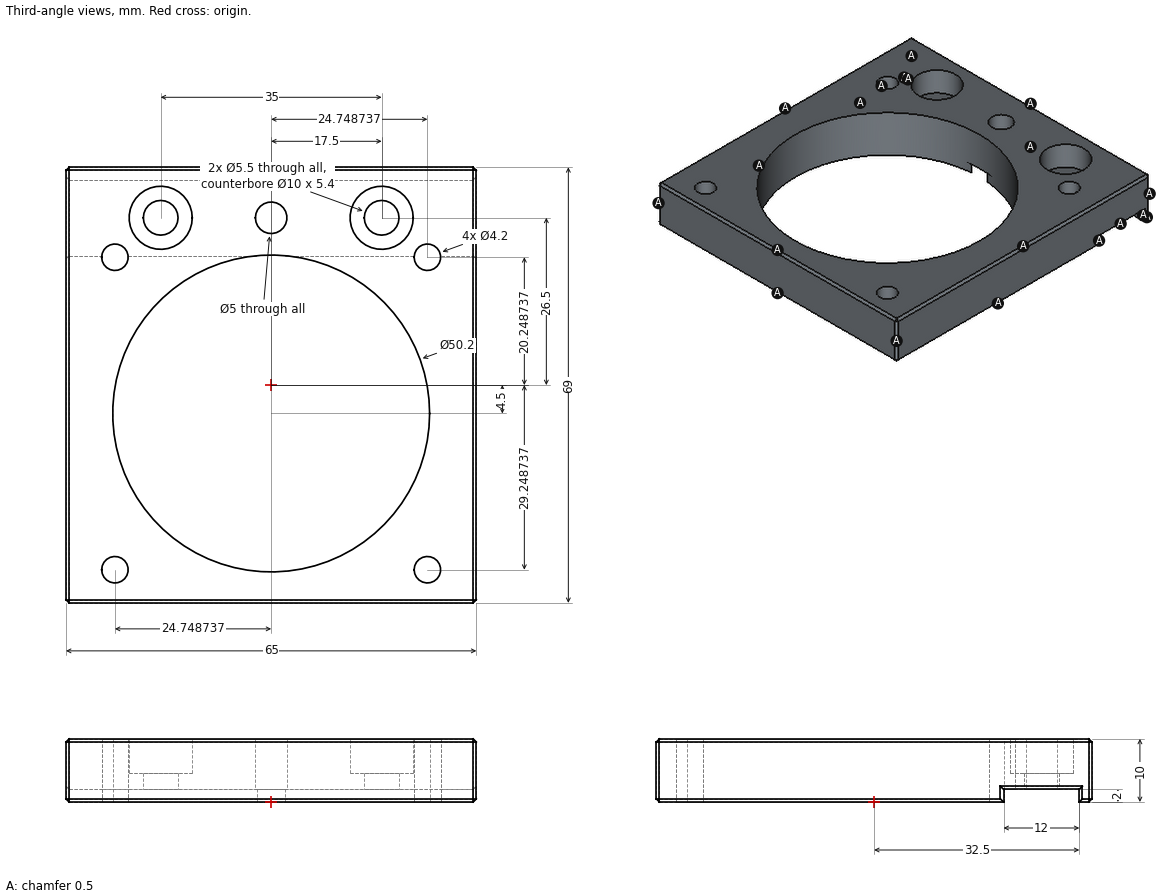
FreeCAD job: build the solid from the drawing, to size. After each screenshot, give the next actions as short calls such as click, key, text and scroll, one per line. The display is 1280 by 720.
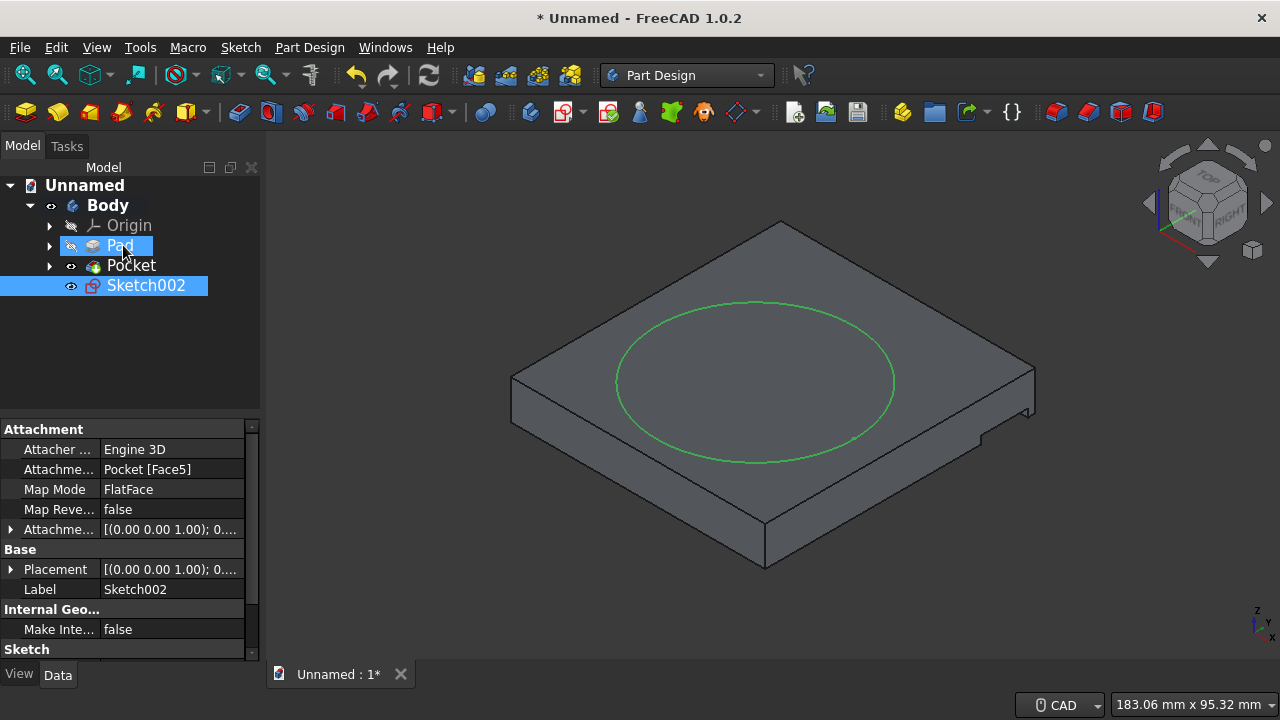
click(240, 112)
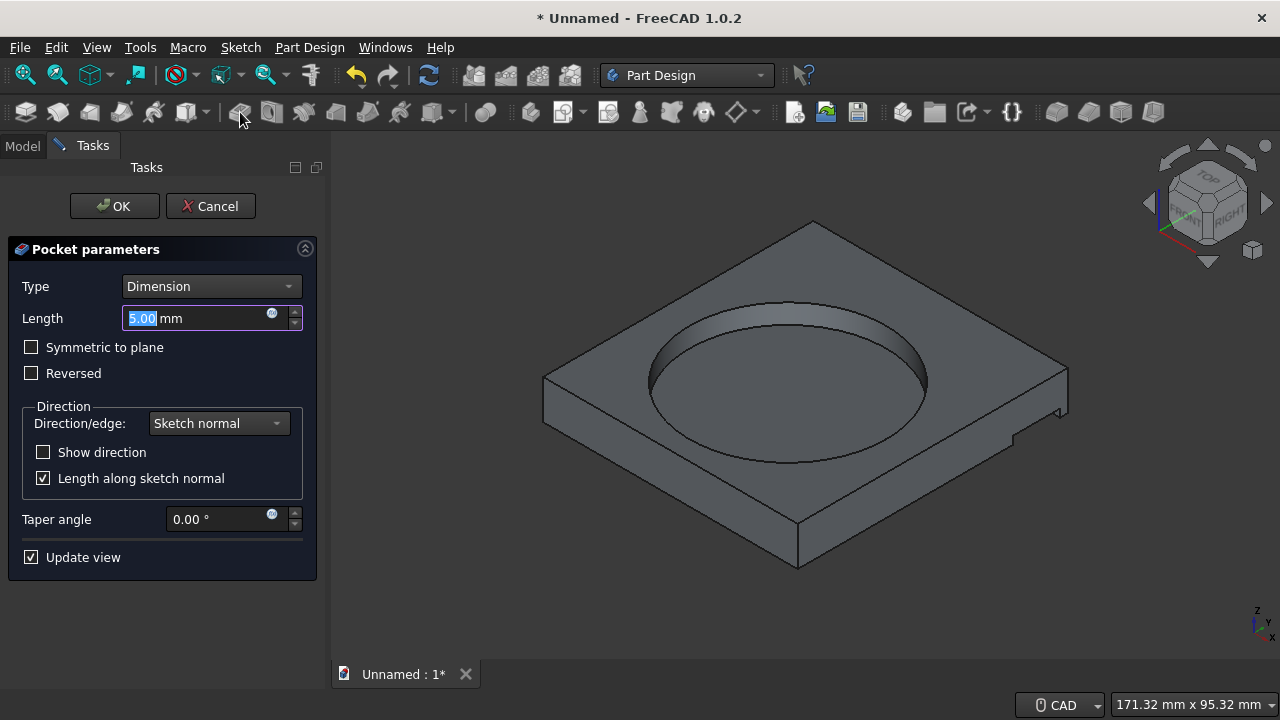
click(212, 286)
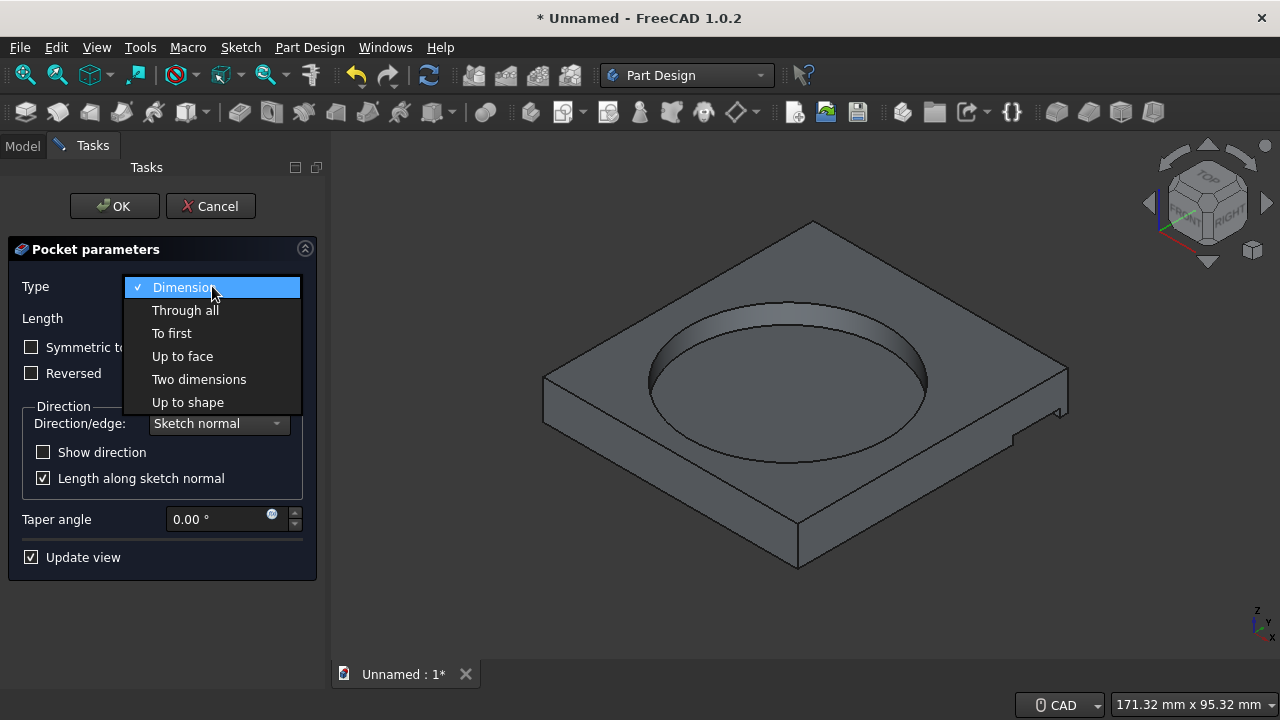
click(212, 310)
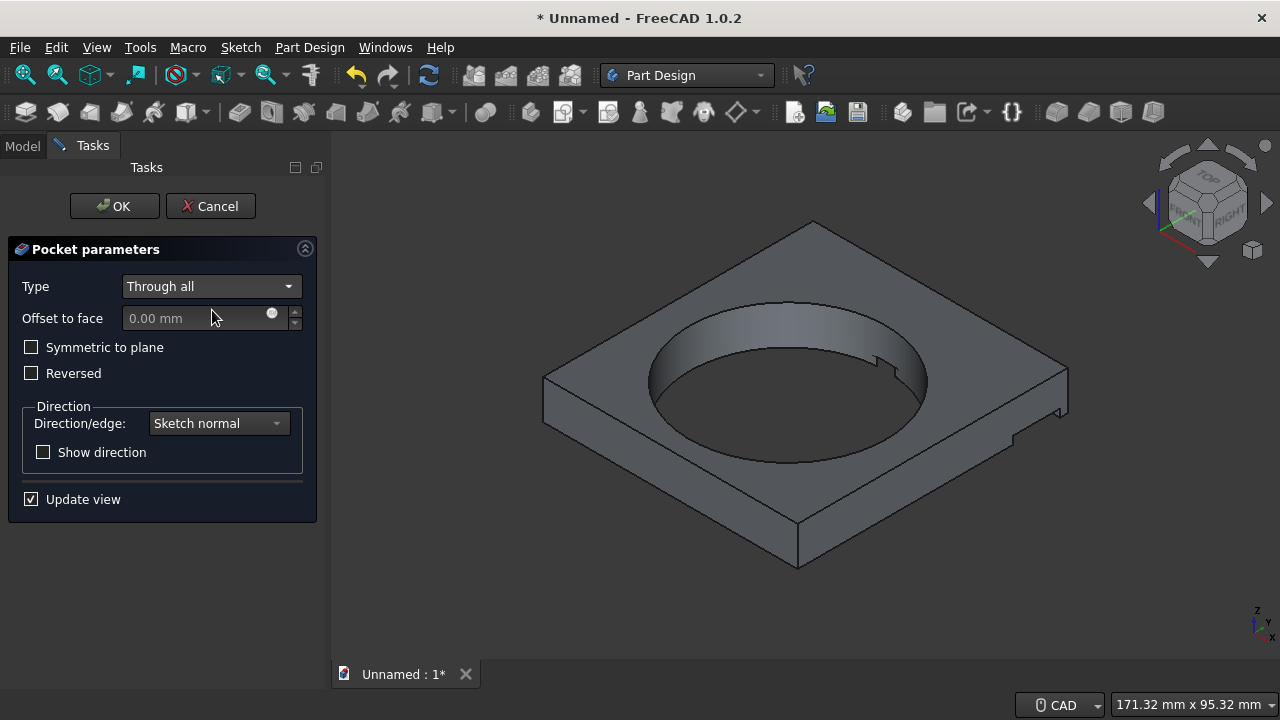
click(115, 206)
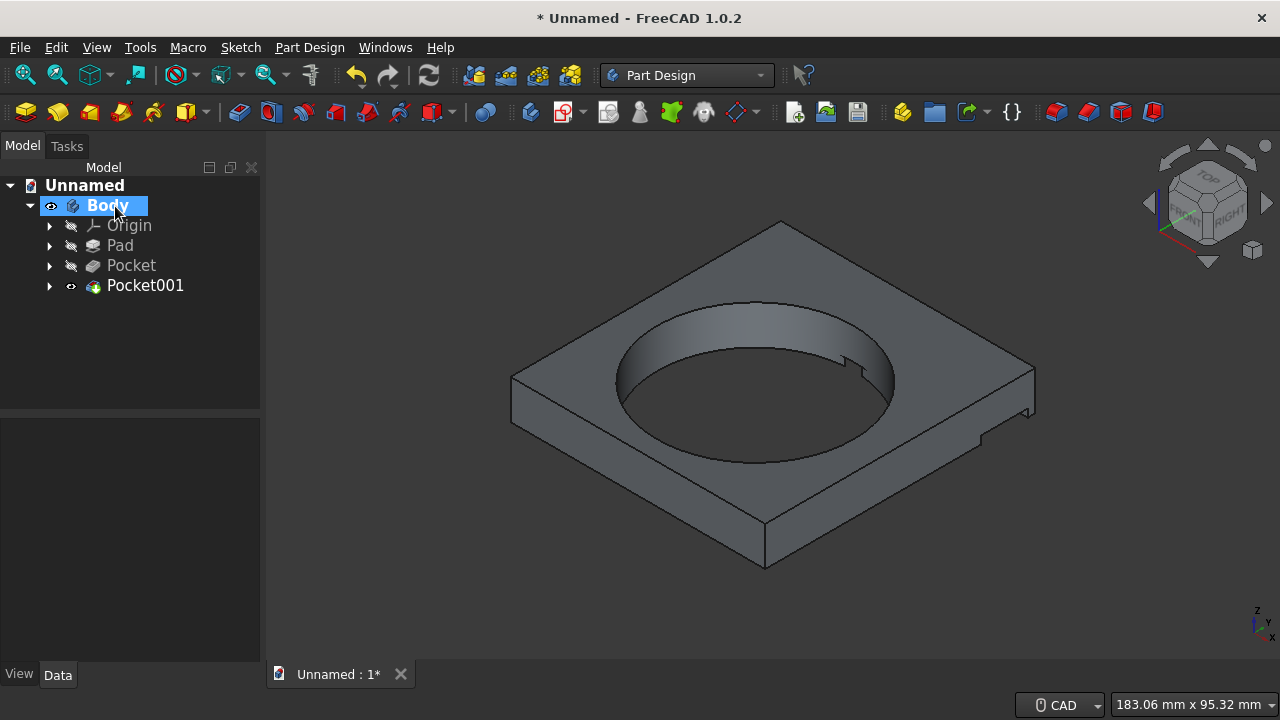
click(923, 369)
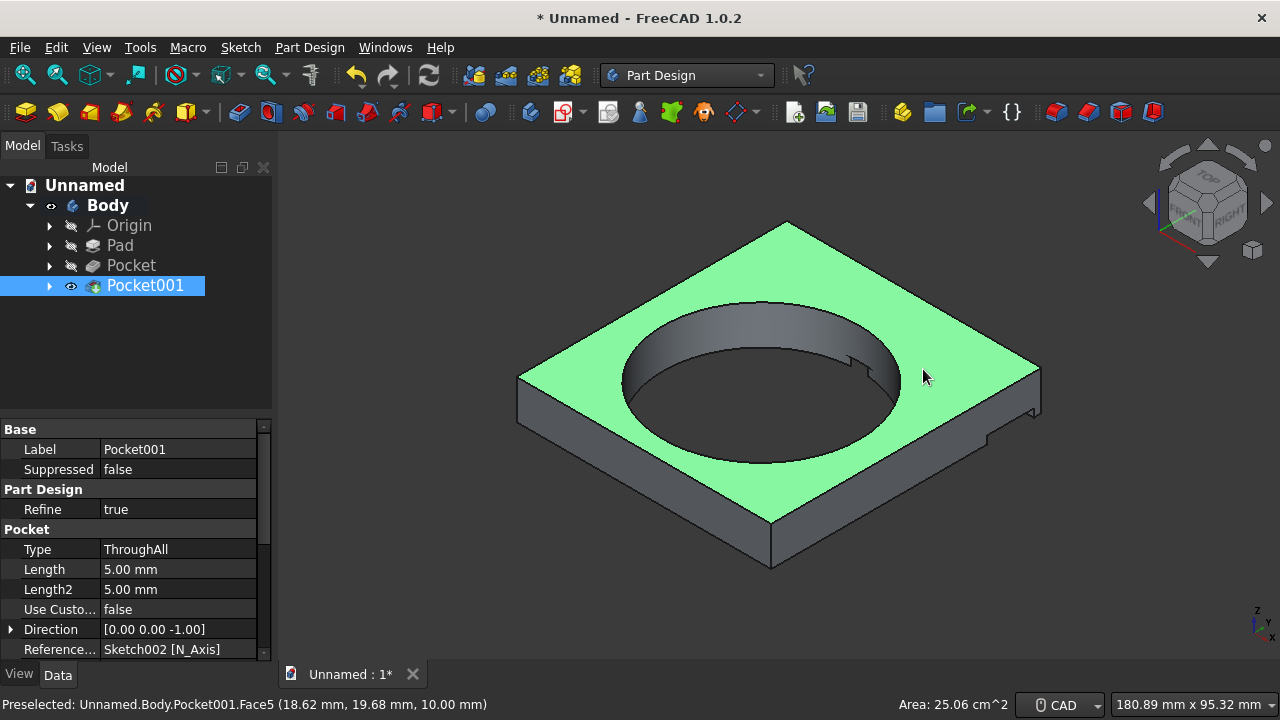
click(564, 112)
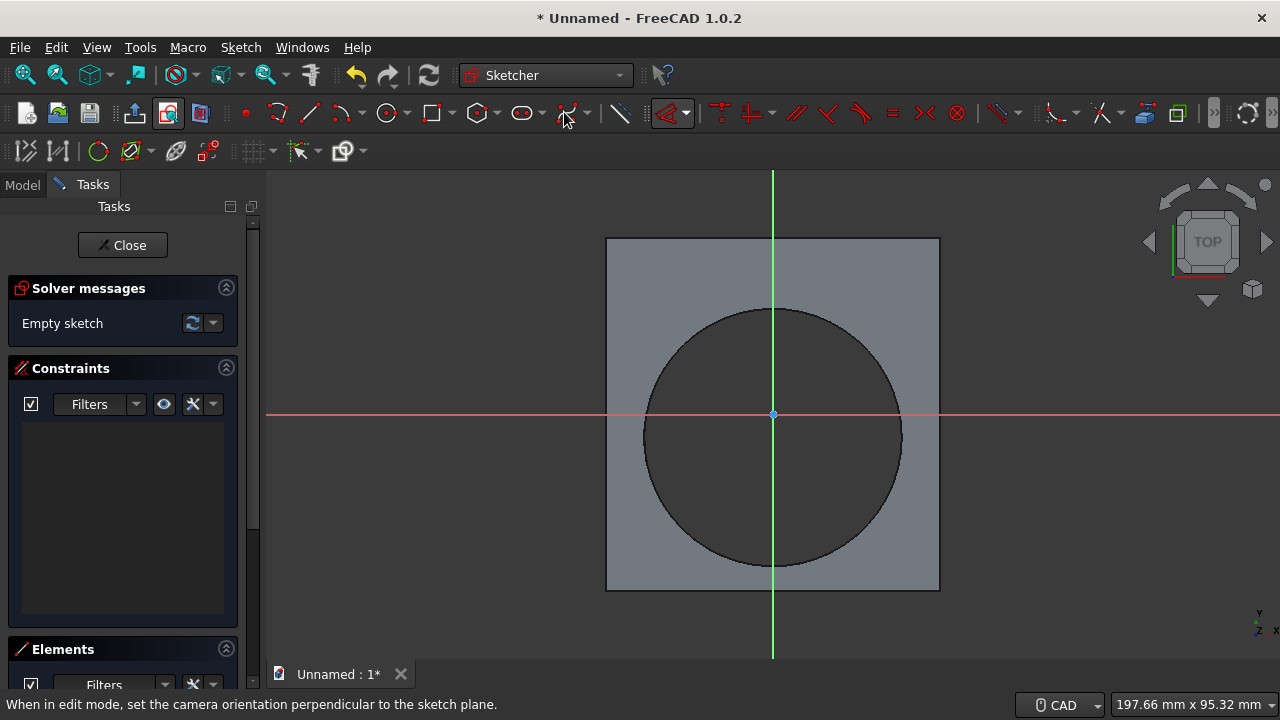
click(388, 114)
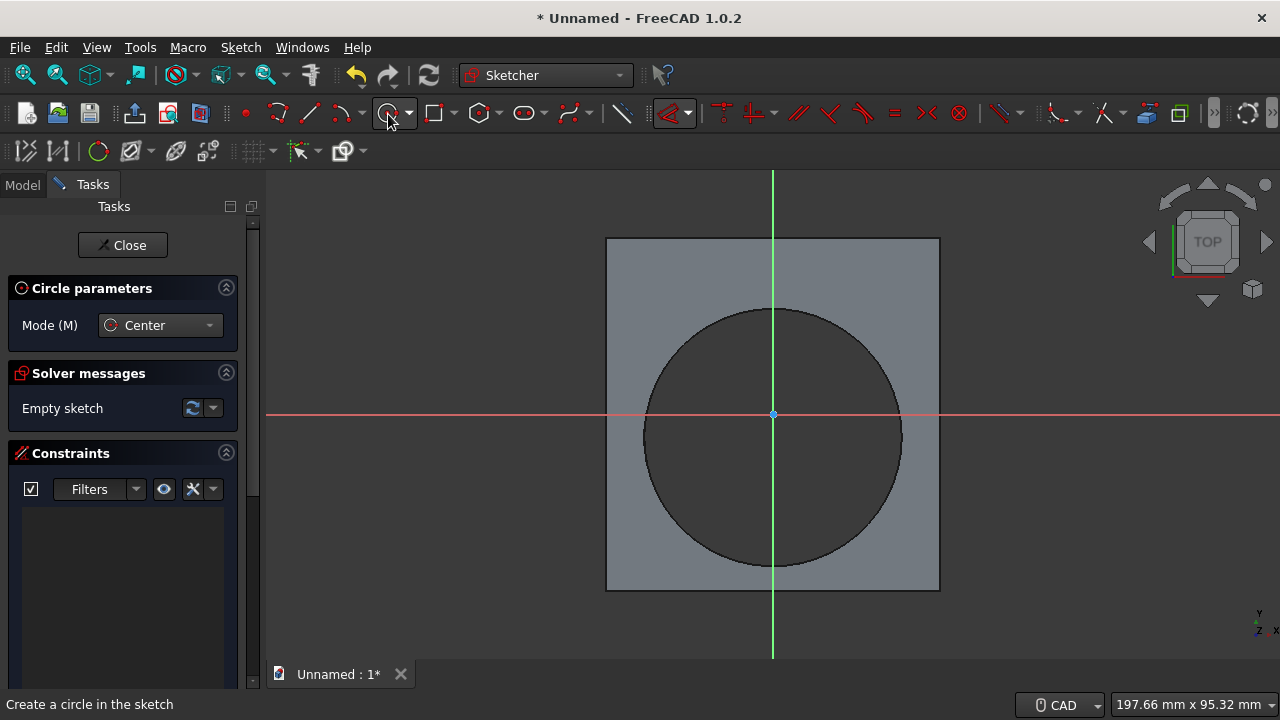
scroll(900, 311, up, 4)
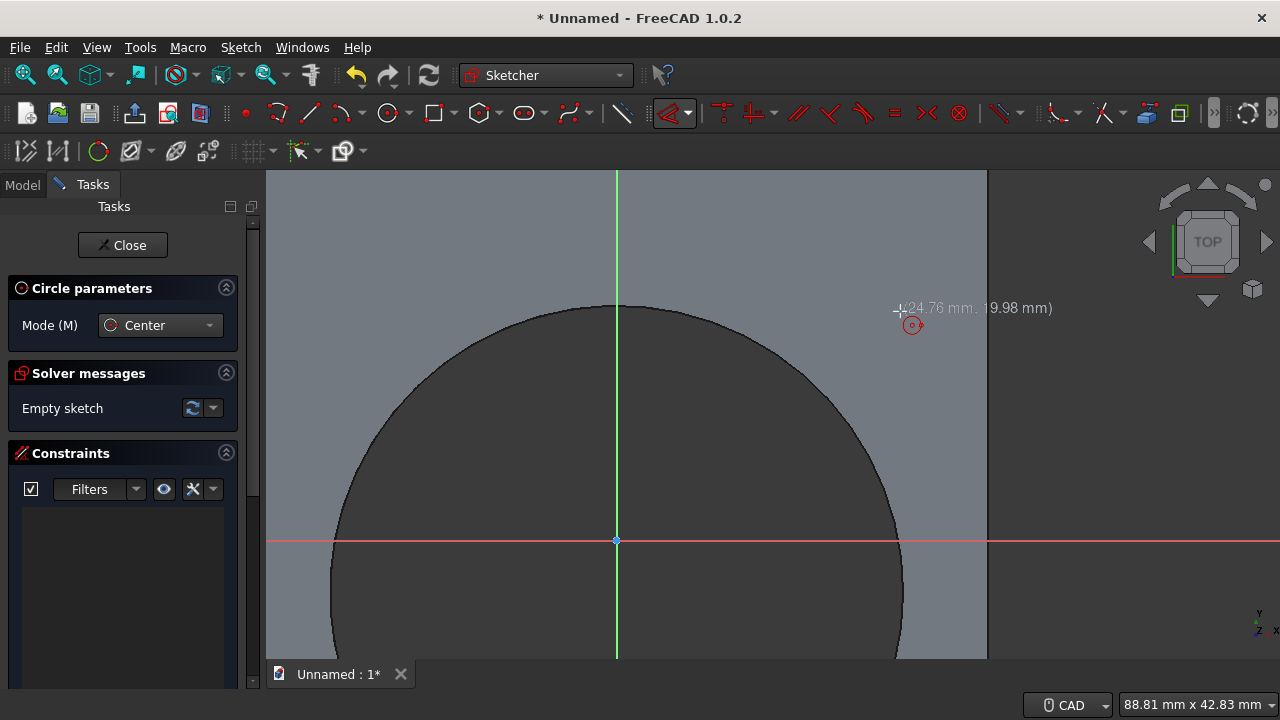
click(899, 310)
click(916, 293)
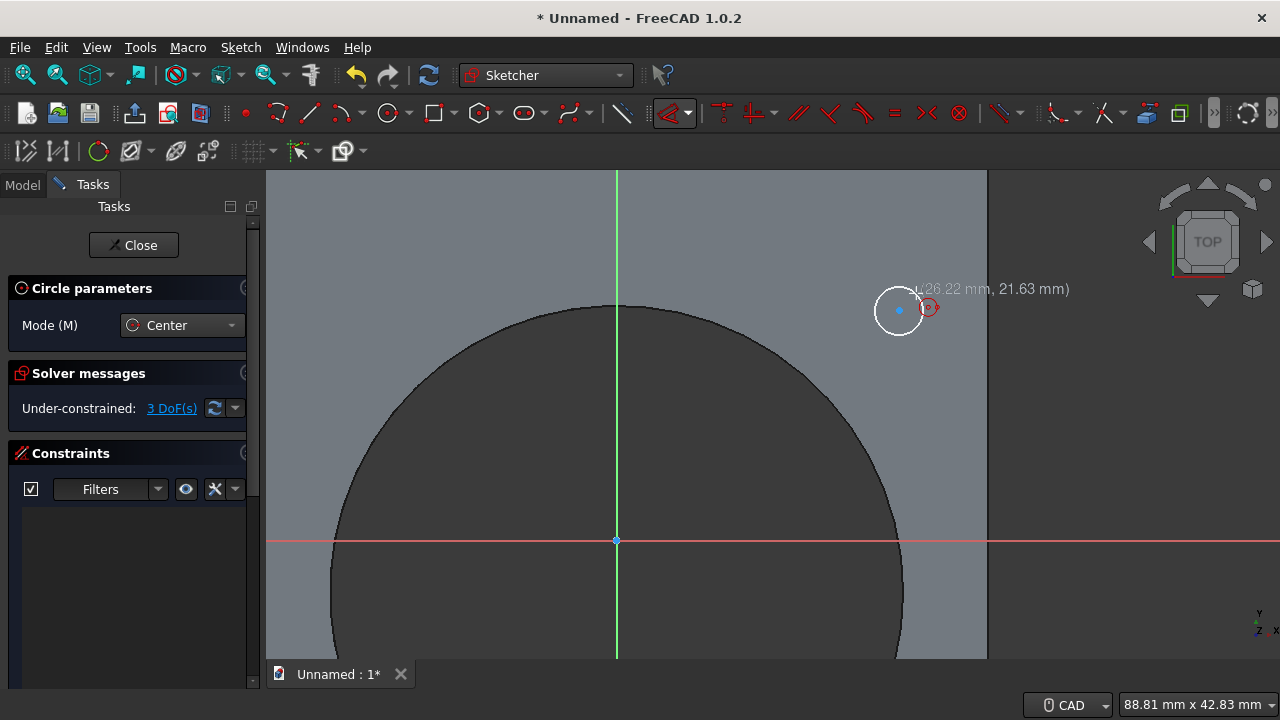
scroll(811, 198, down, 3)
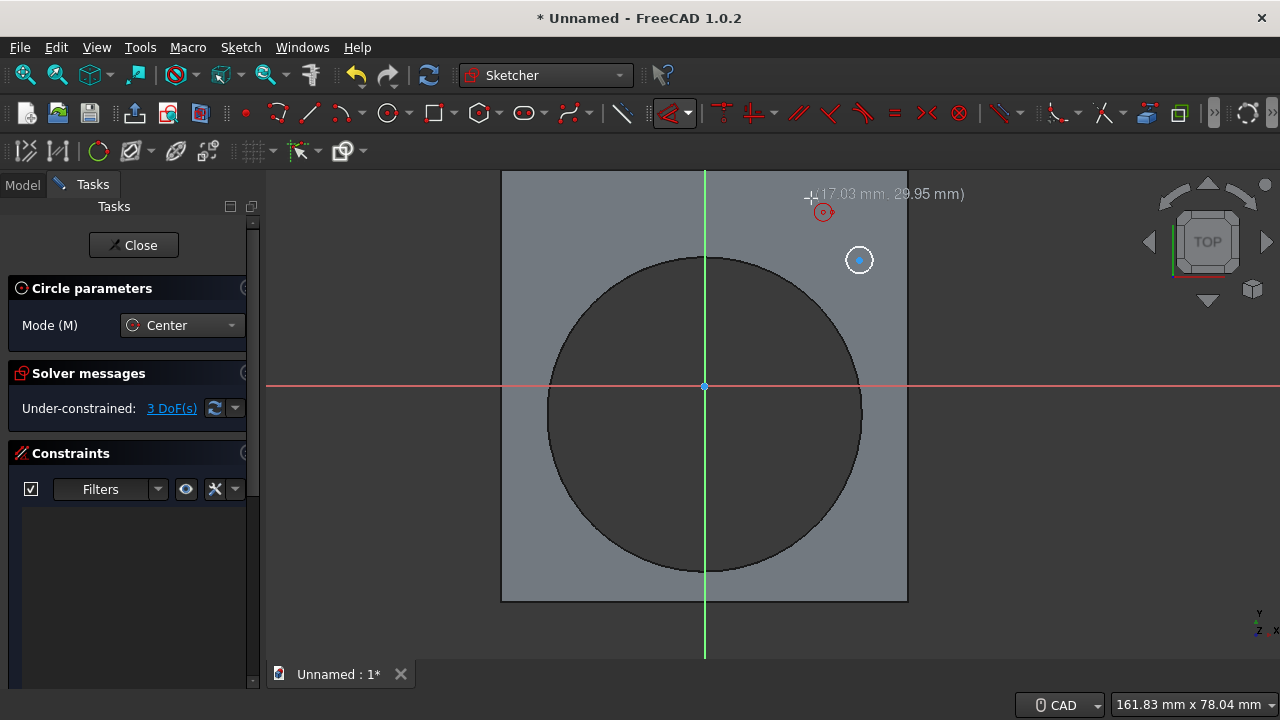
scroll(860, 570, up, 3)